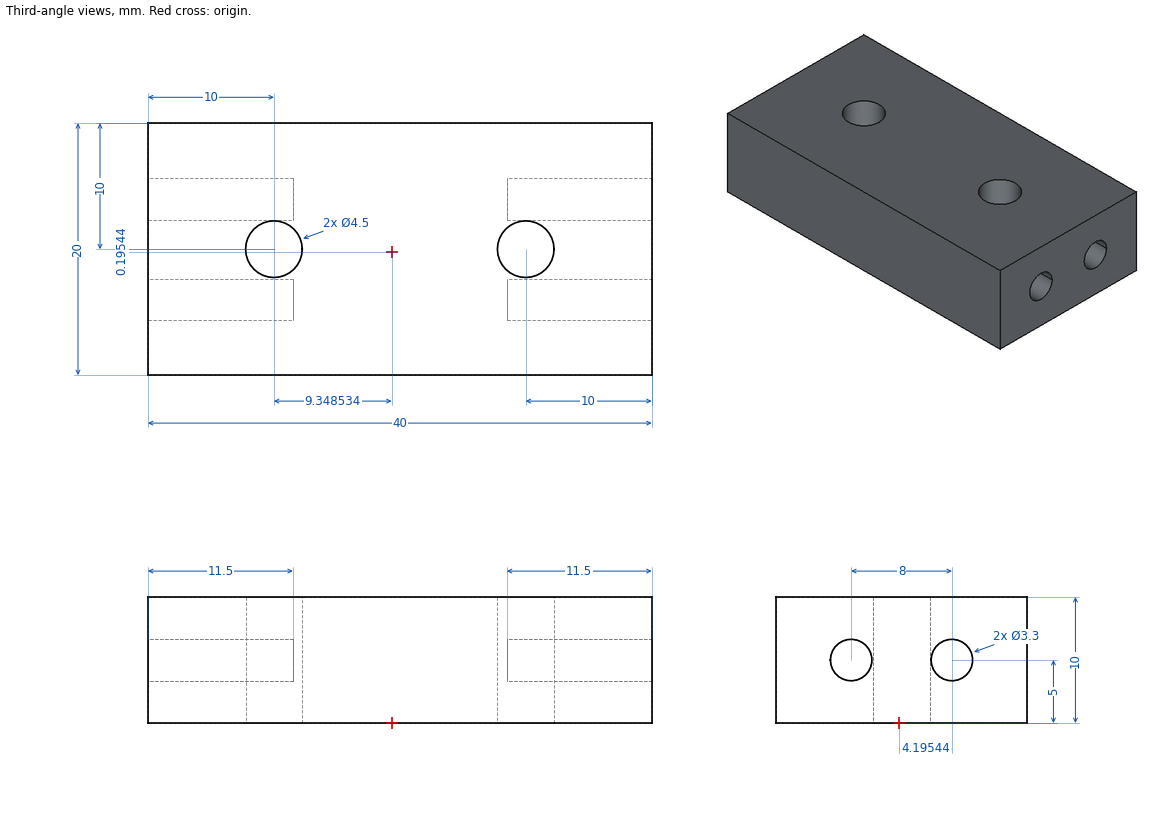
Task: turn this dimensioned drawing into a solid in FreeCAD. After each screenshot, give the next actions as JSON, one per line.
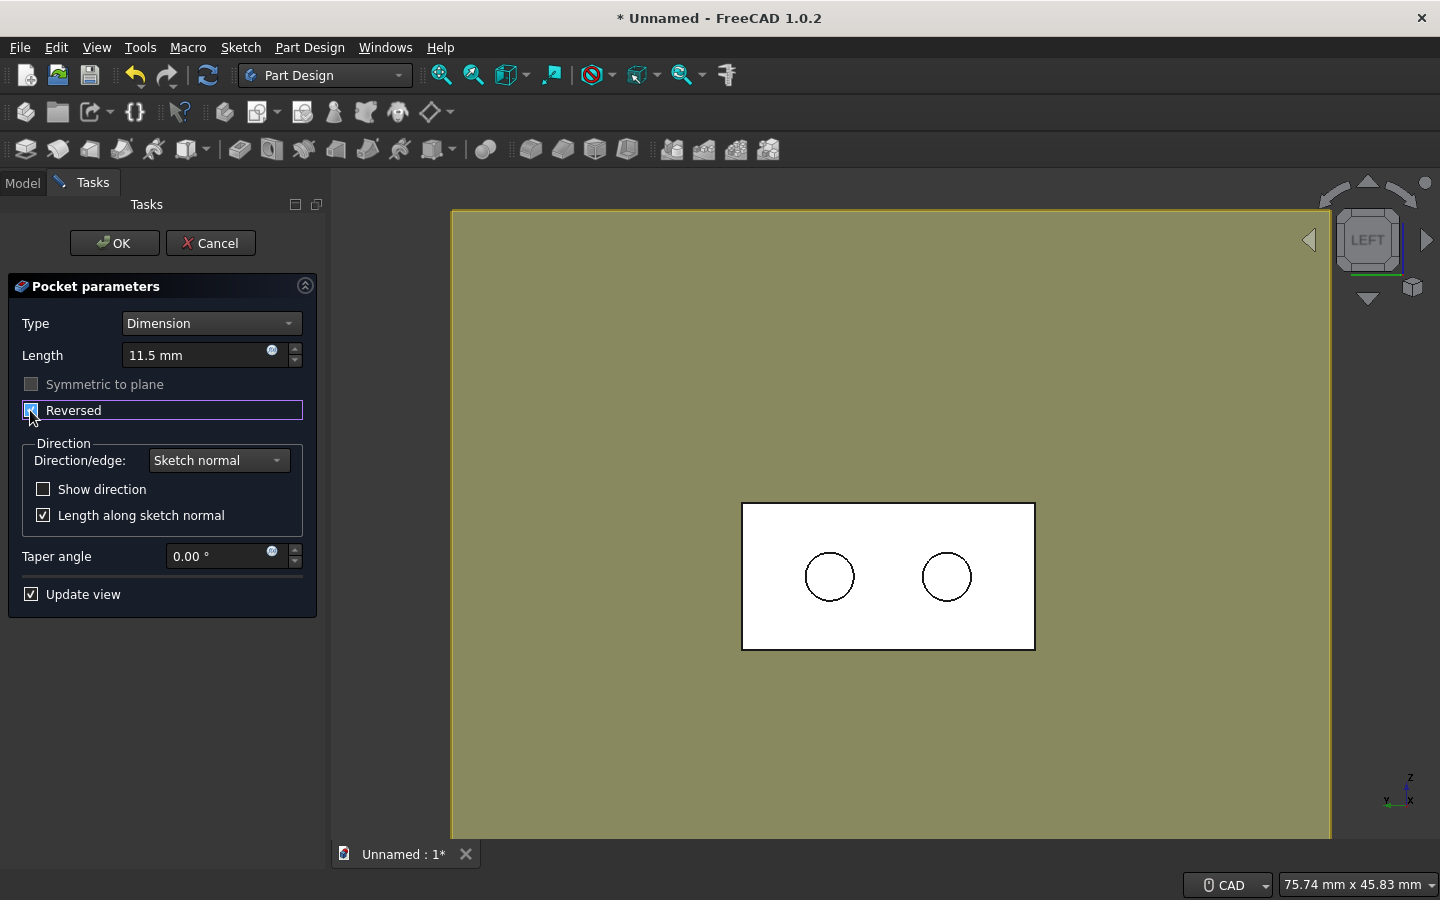
{"action": "left_click", "coordinate": [115, 243]}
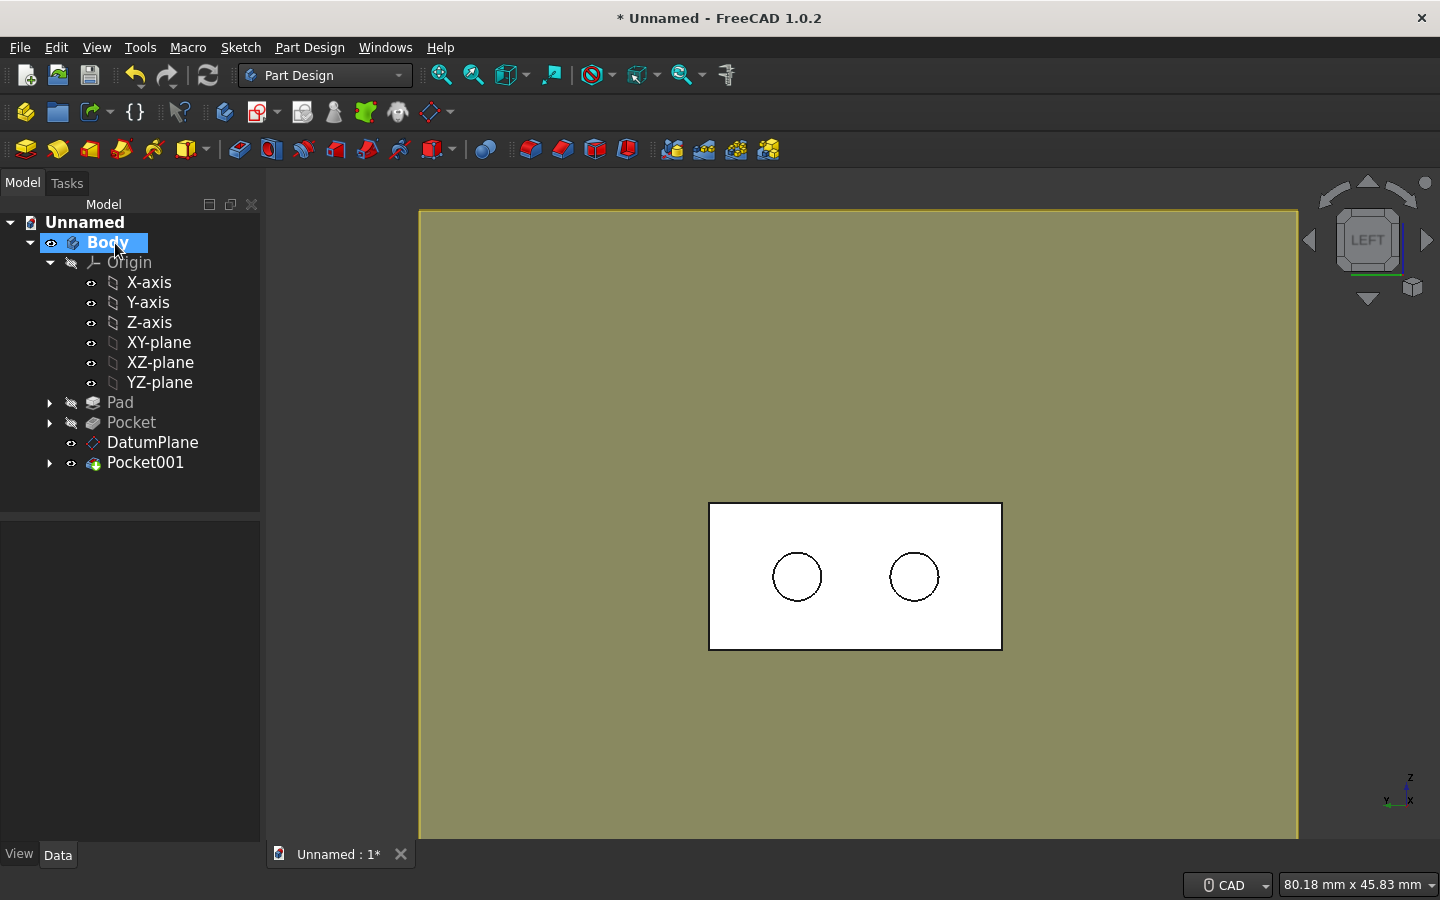
{"action": "left_click", "coordinate": [116, 443]}
{"action": "key", "text": "space"}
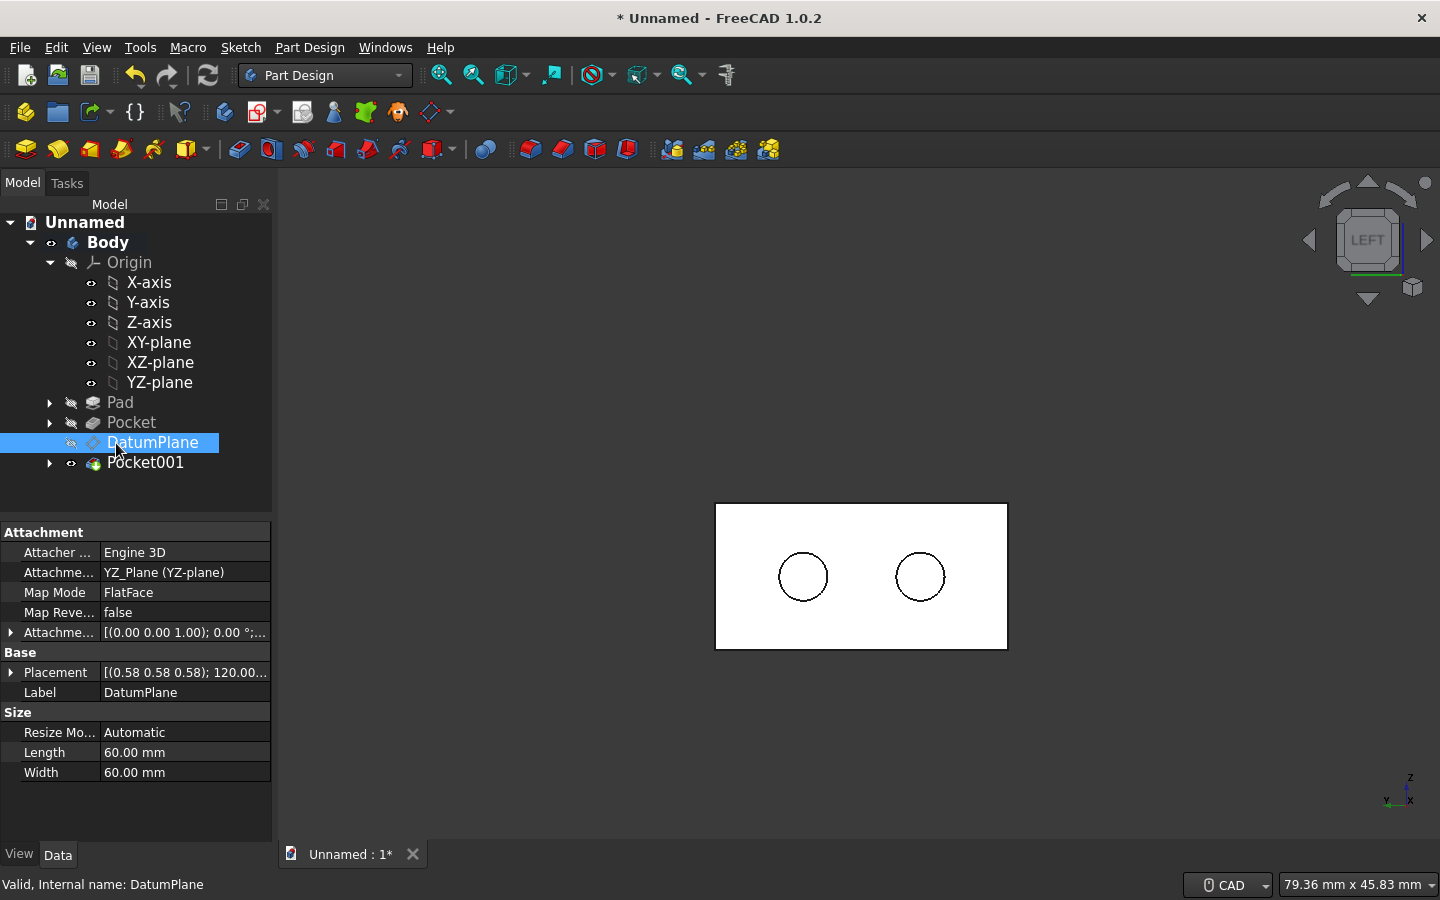
{"action": "key", "text": "0"}